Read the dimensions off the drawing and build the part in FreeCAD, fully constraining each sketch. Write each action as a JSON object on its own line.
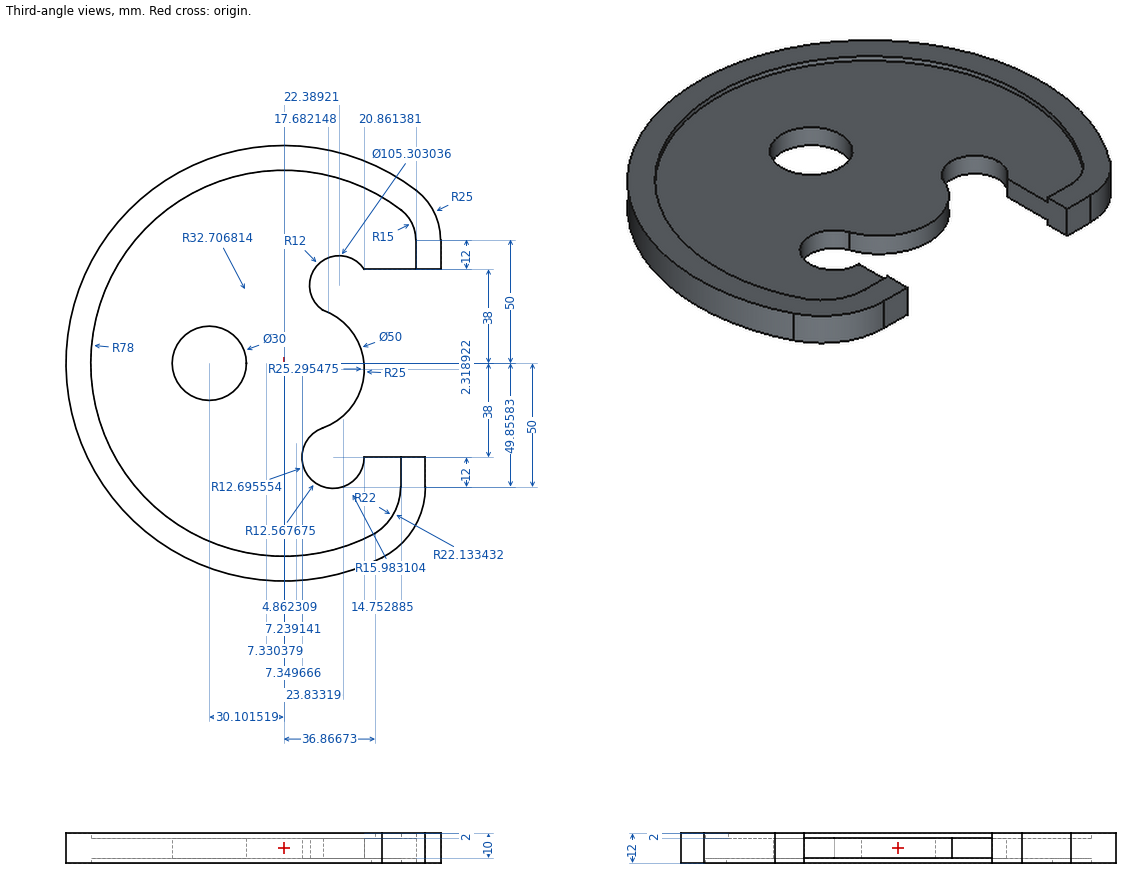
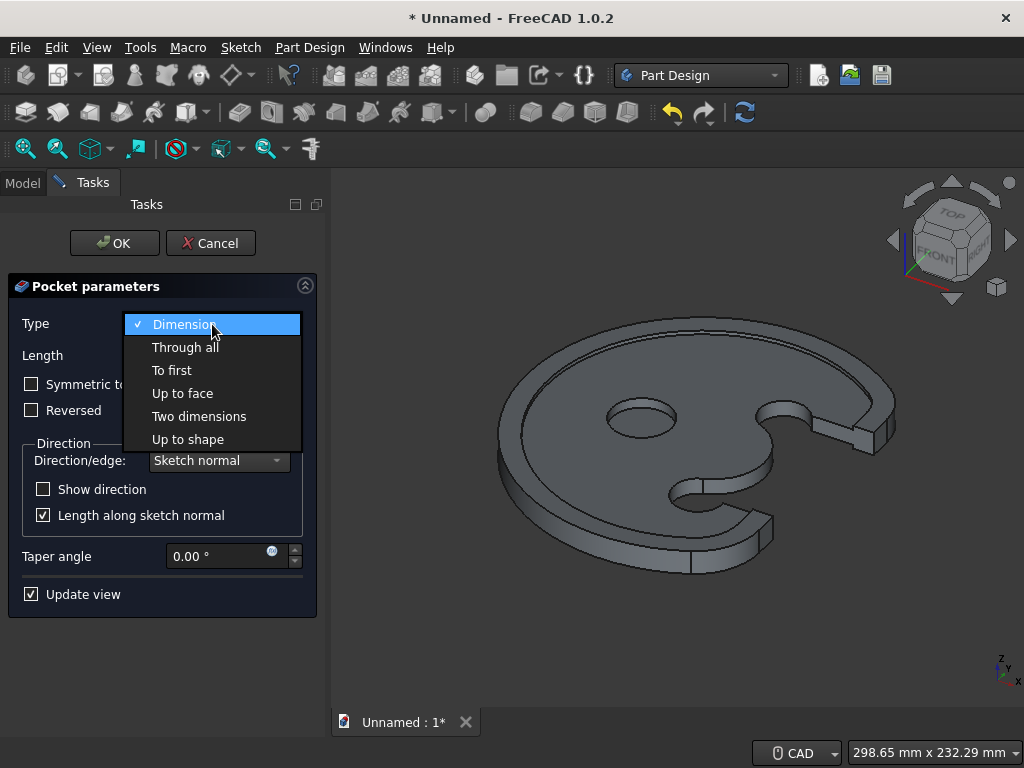
{"action": "left_click", "coordinate": [212, 348]}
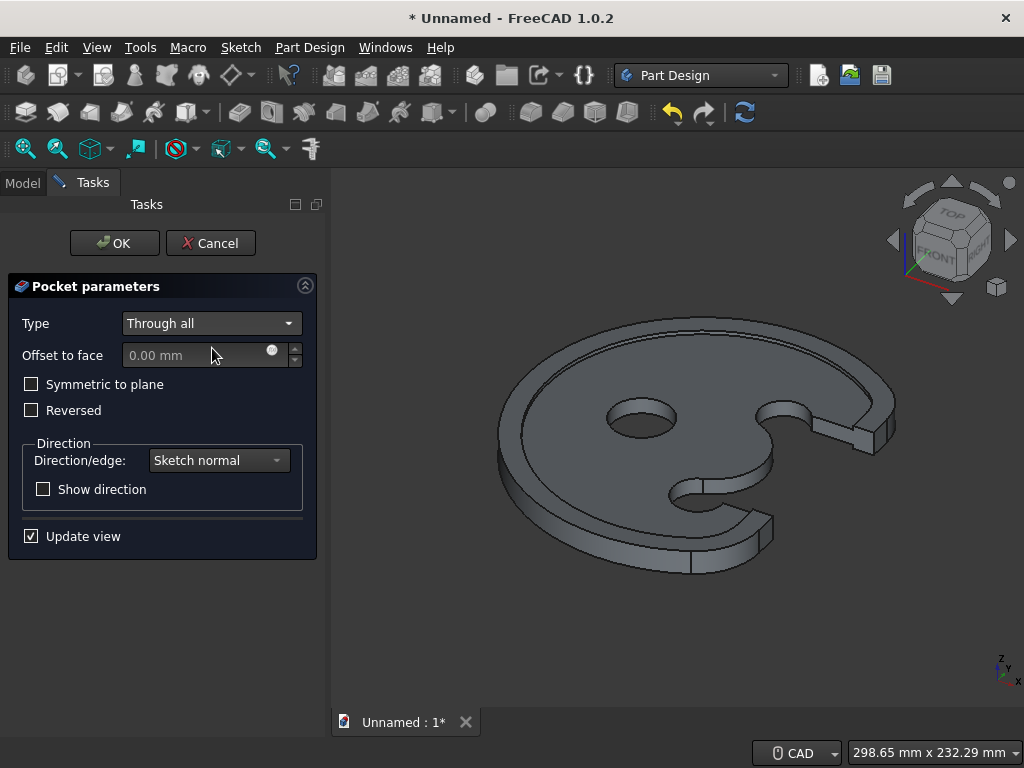
{"action": "left_click", "coordinate": [115, 243]}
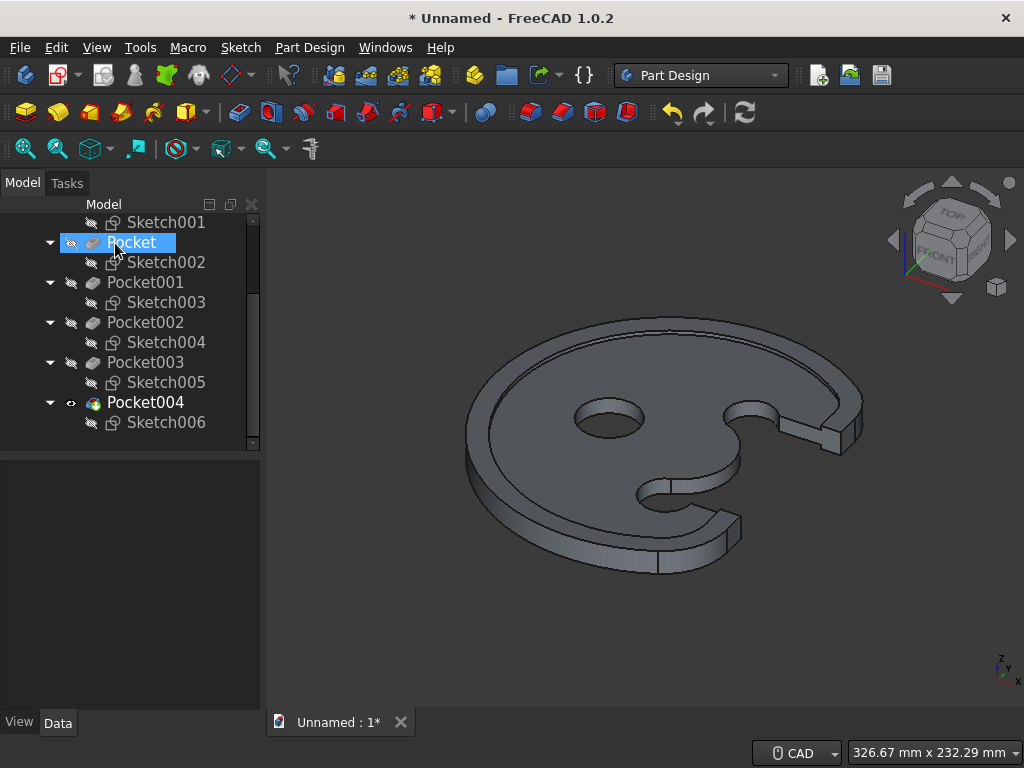
{"action": "key", "text": "0"}